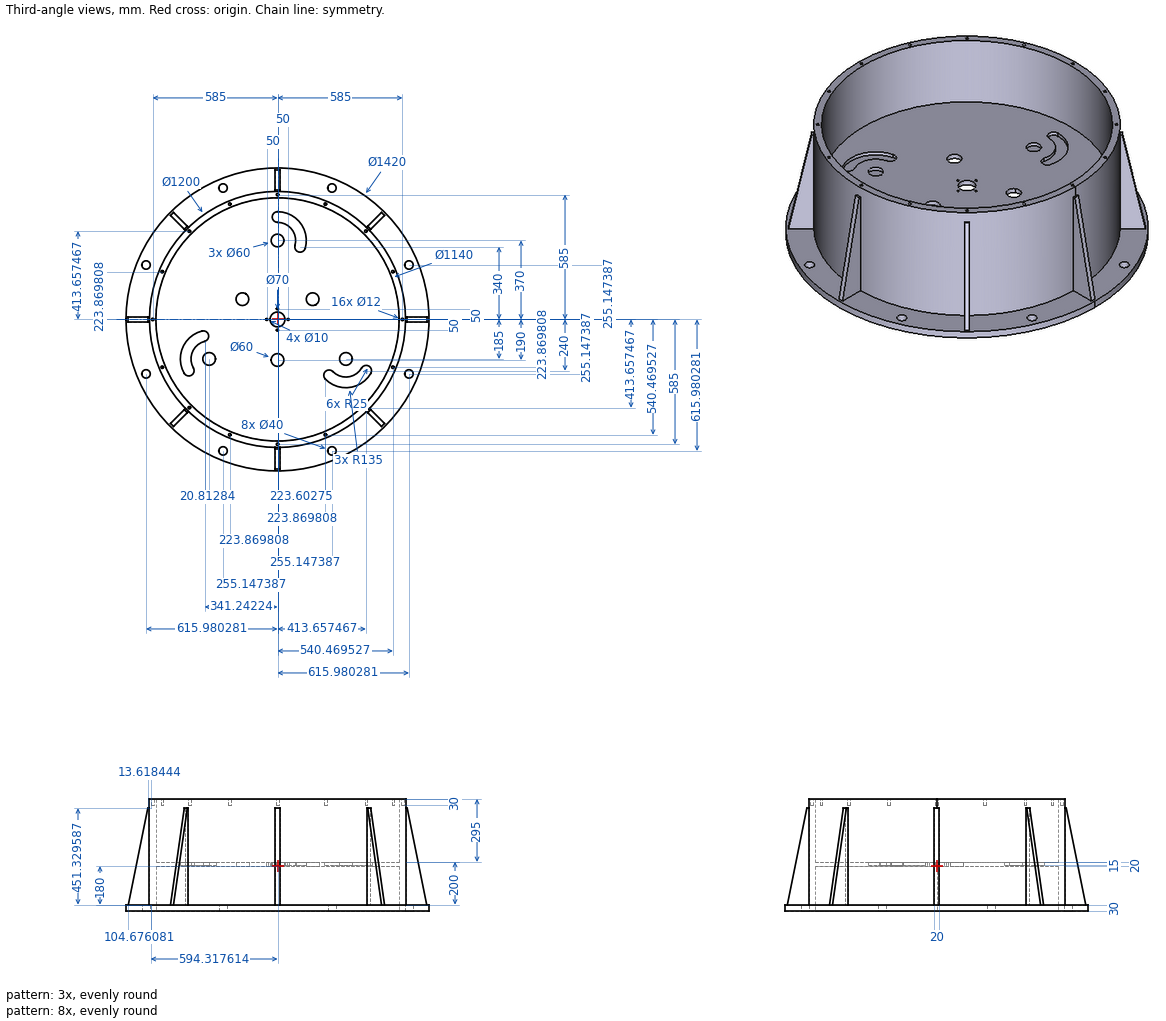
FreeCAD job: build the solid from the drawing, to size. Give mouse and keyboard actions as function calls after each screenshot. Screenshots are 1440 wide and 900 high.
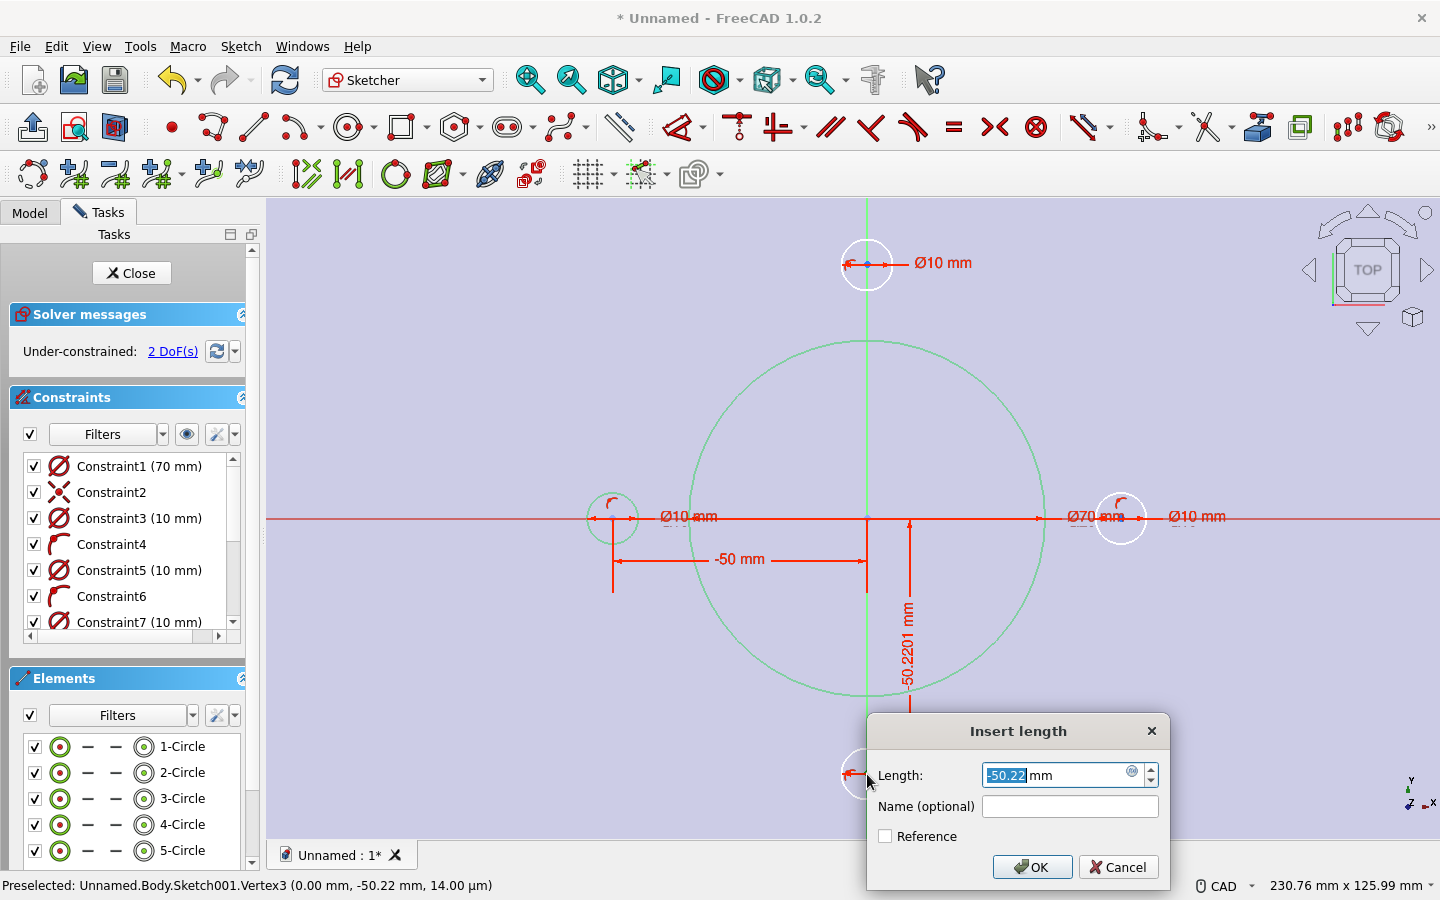
text(-50)
key(Return)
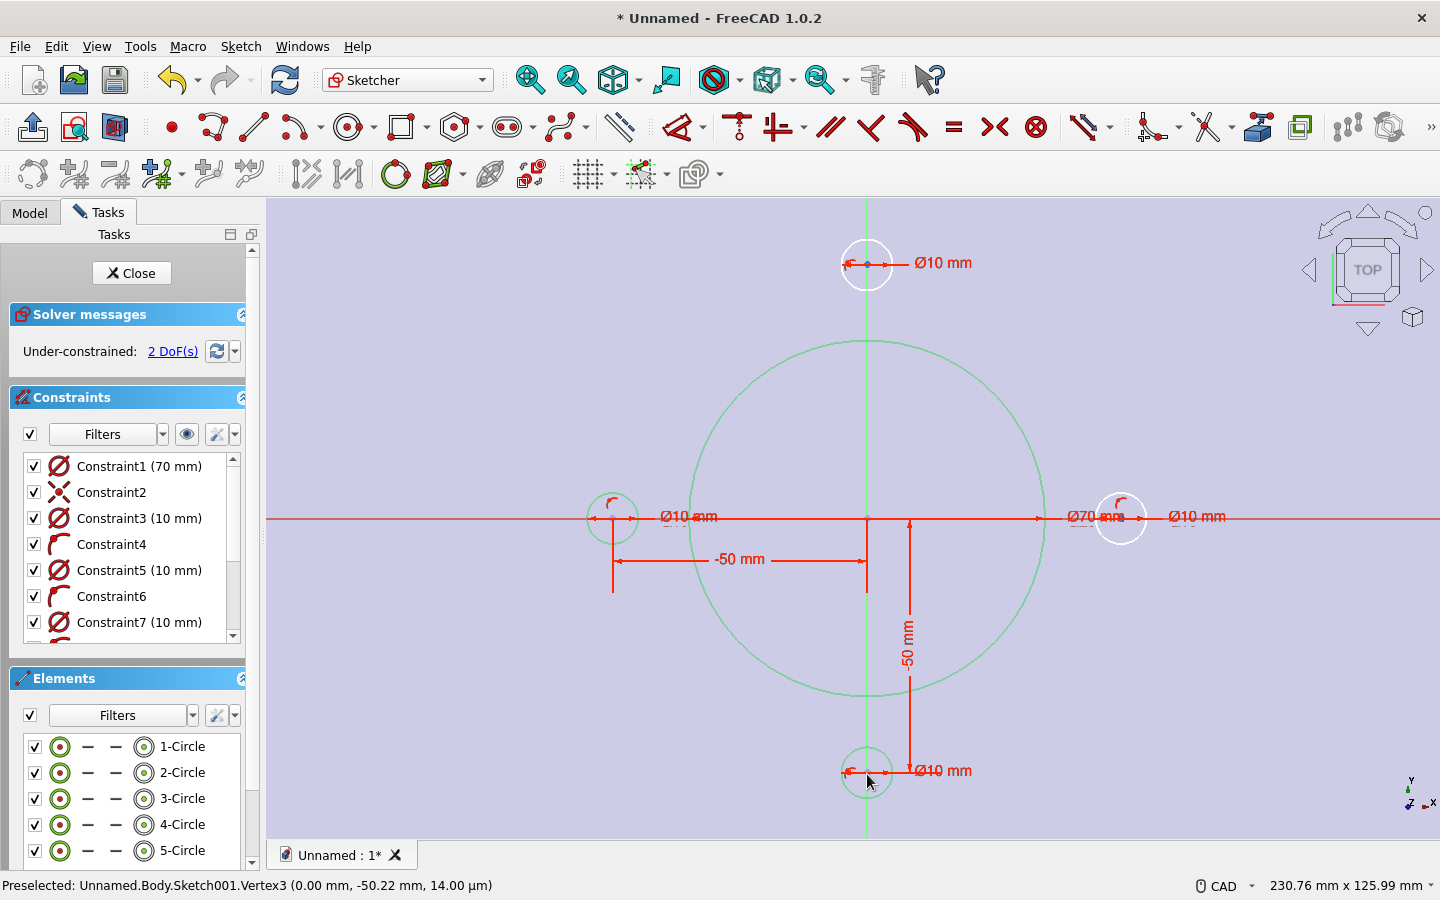
click(1121, 518)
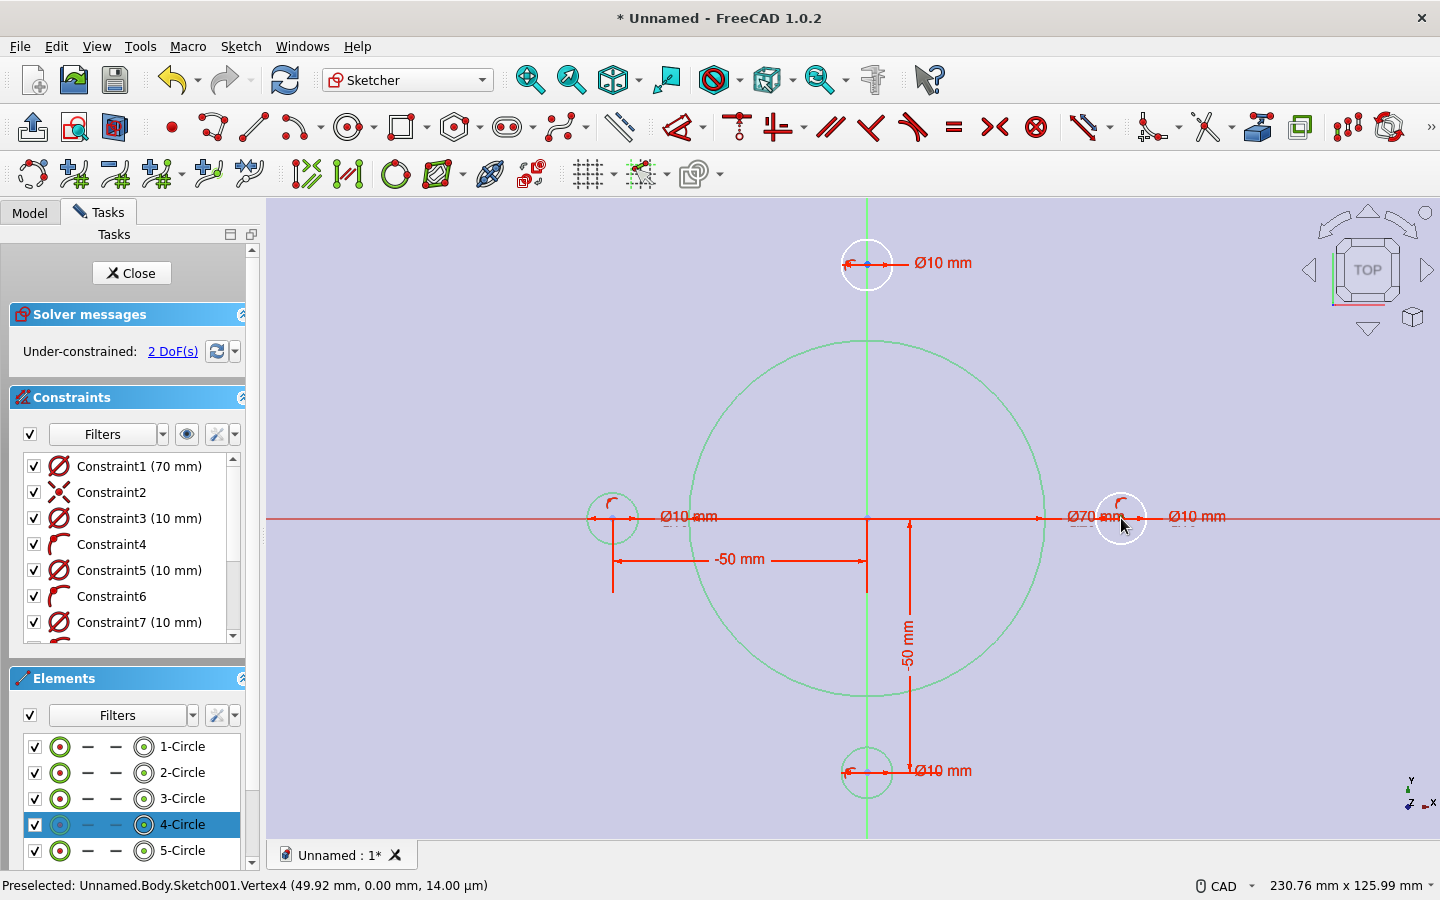
key(l)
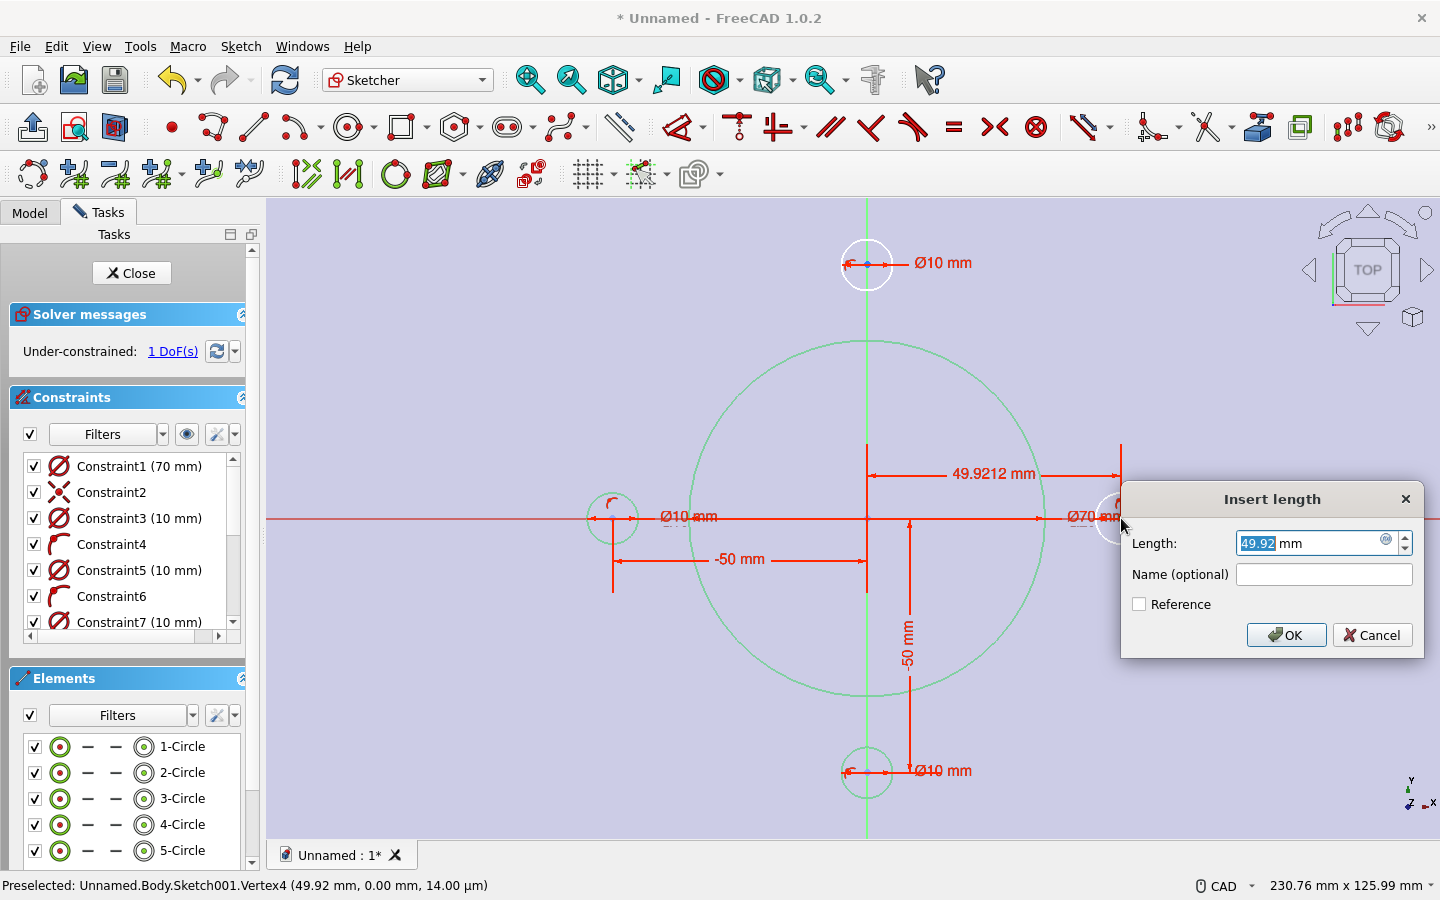
text(50)
key(Return)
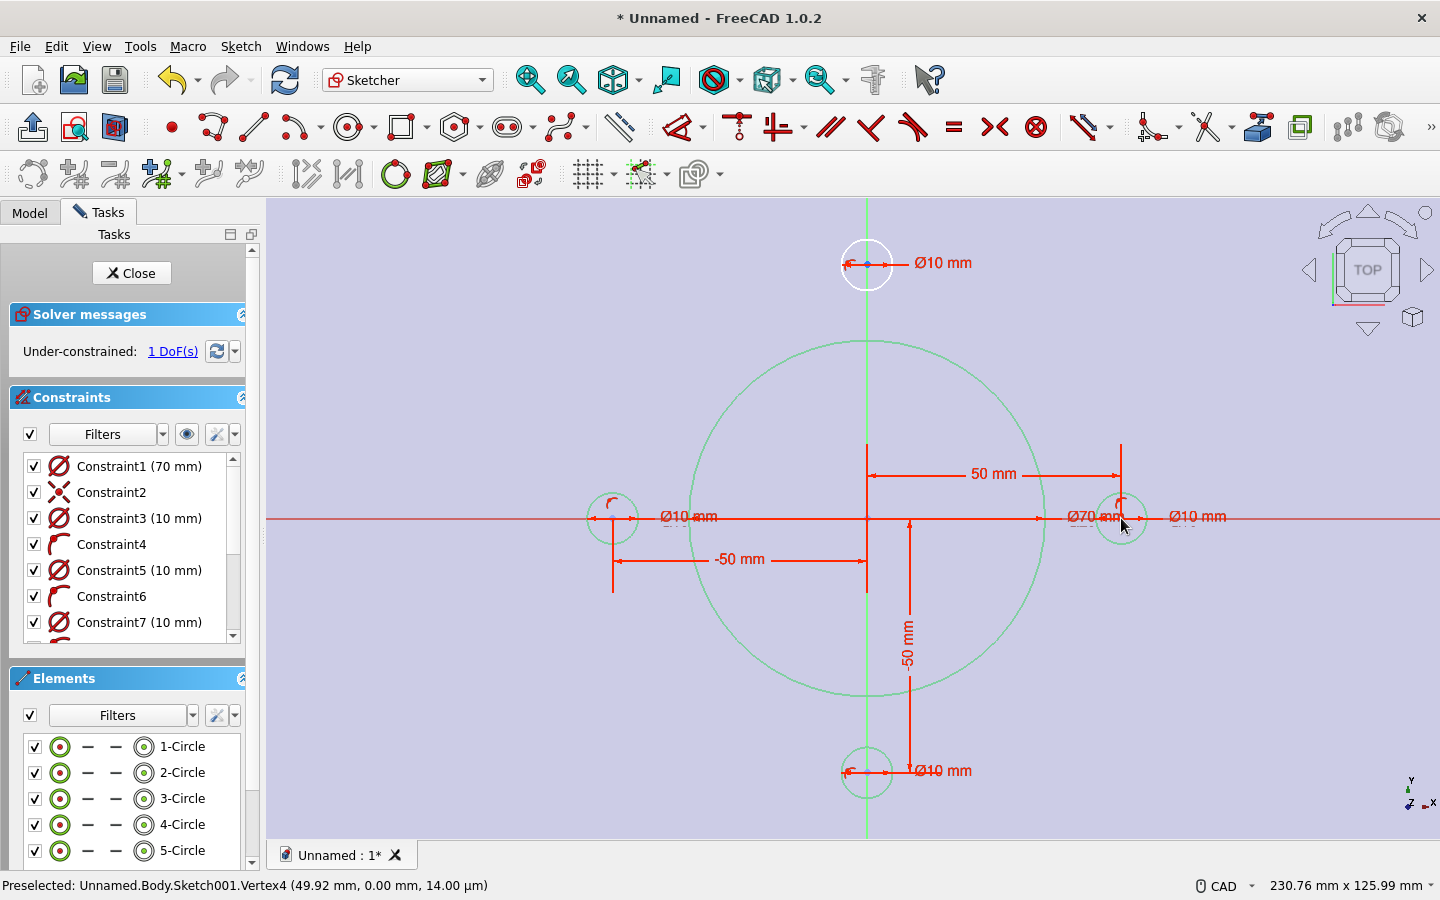
click(867, 265)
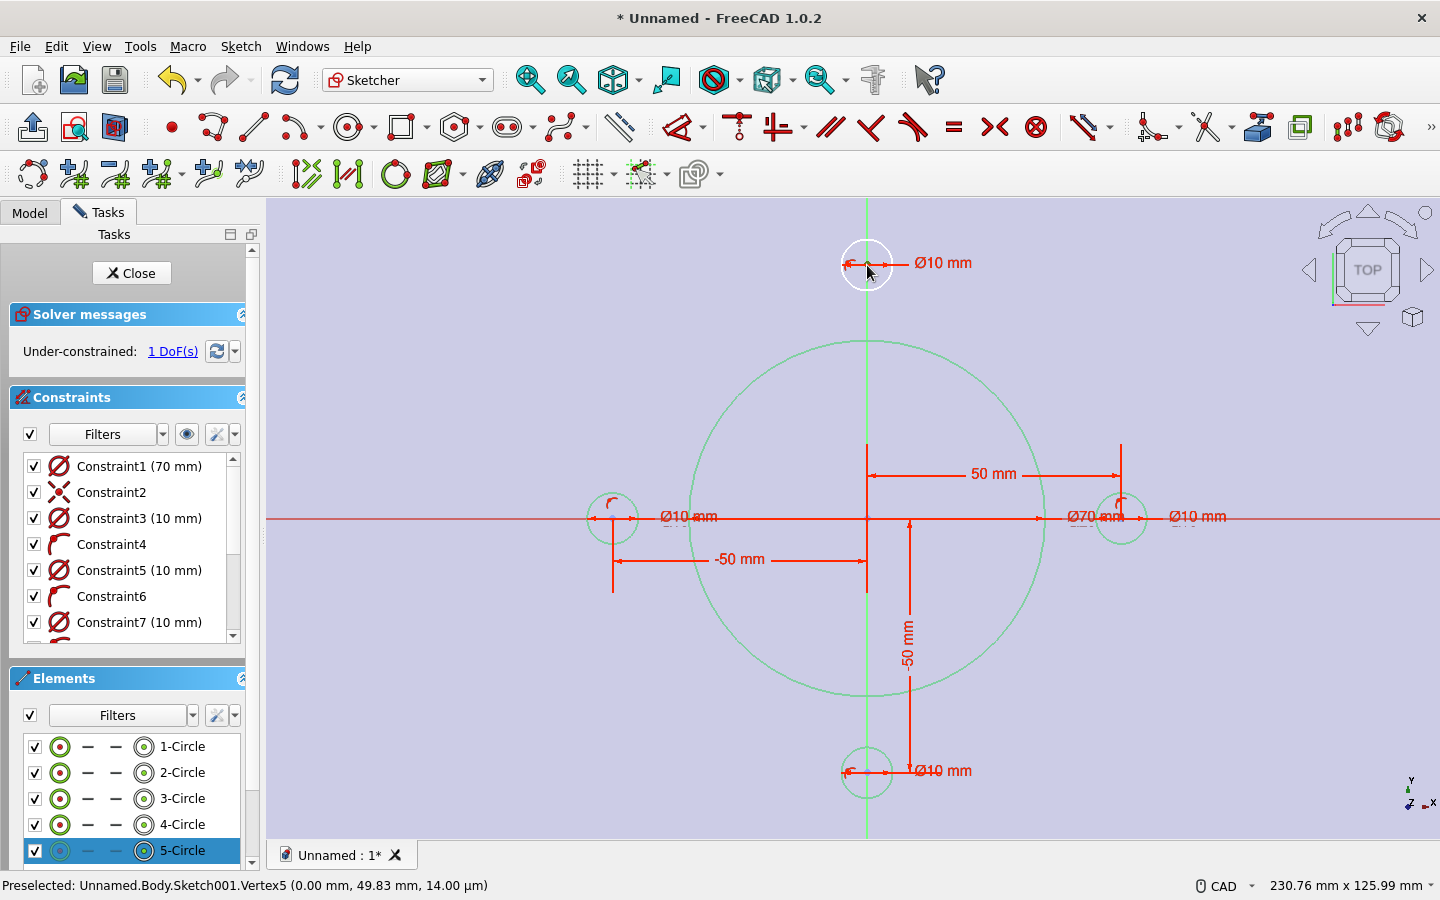
key(i)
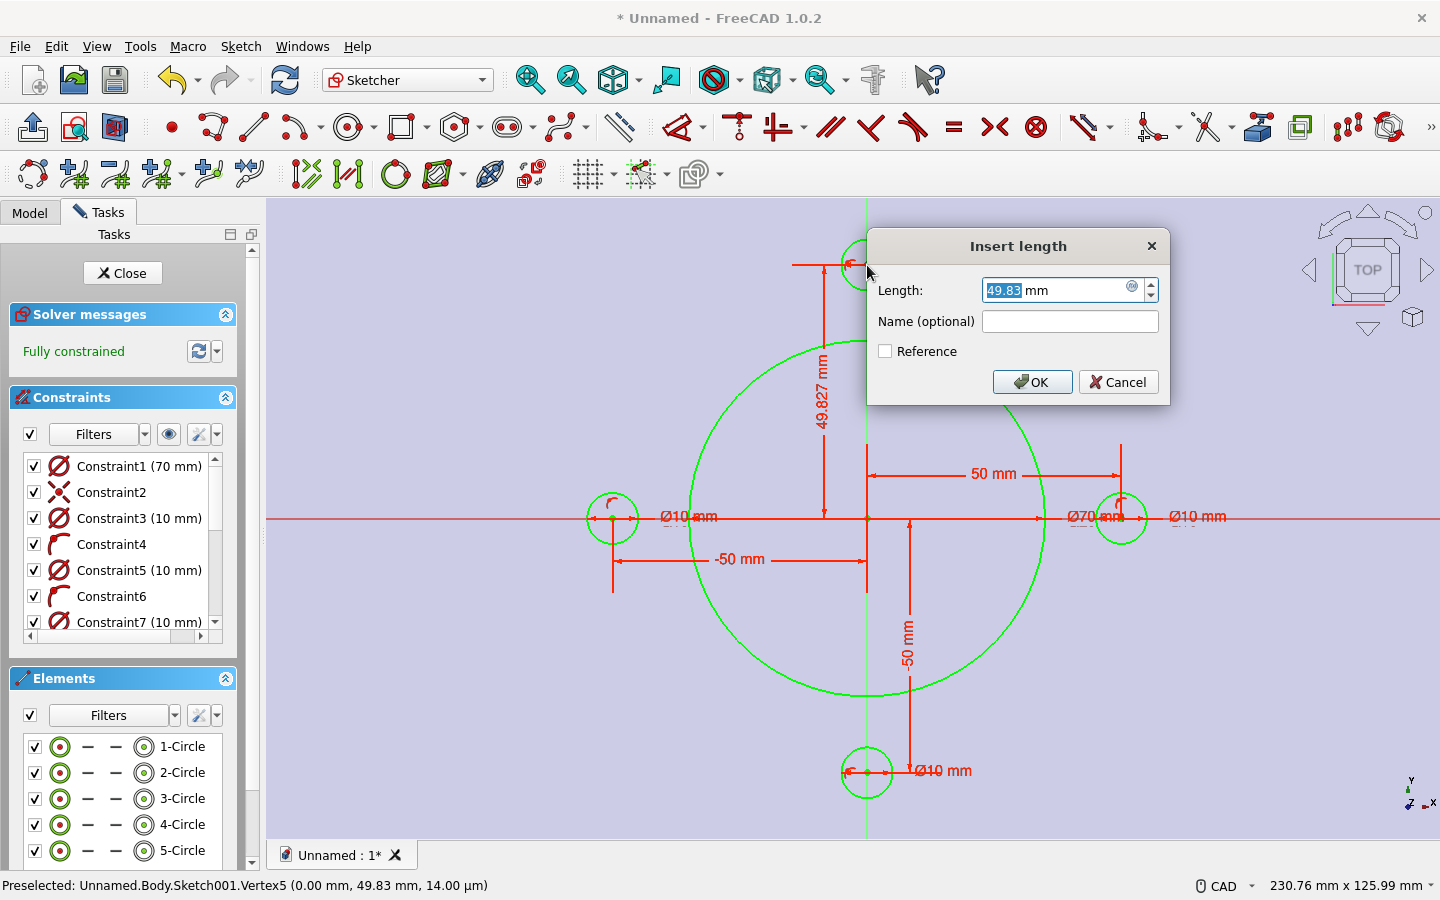
text(50)
key(Return)